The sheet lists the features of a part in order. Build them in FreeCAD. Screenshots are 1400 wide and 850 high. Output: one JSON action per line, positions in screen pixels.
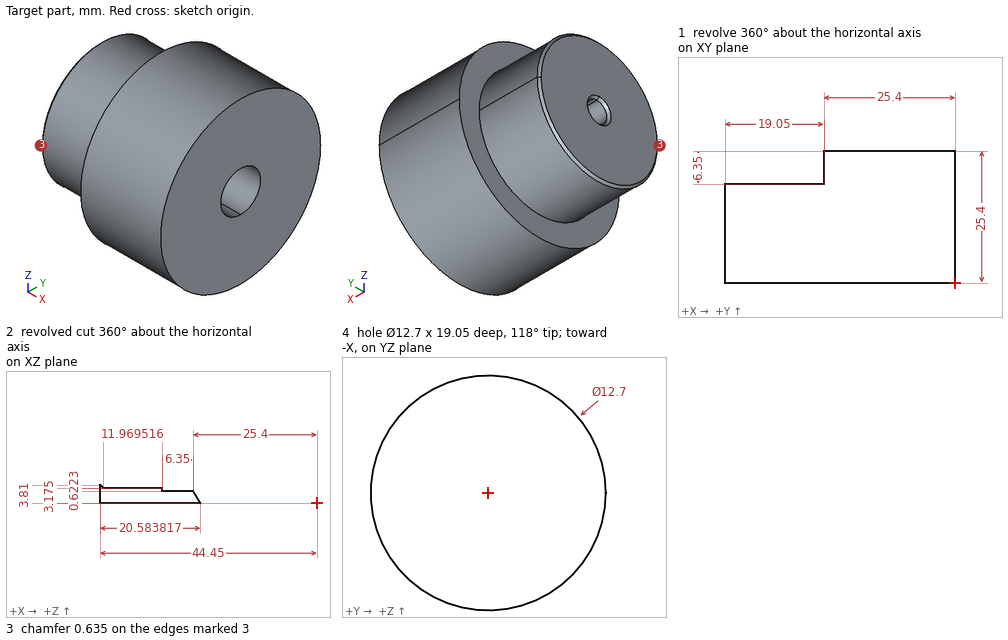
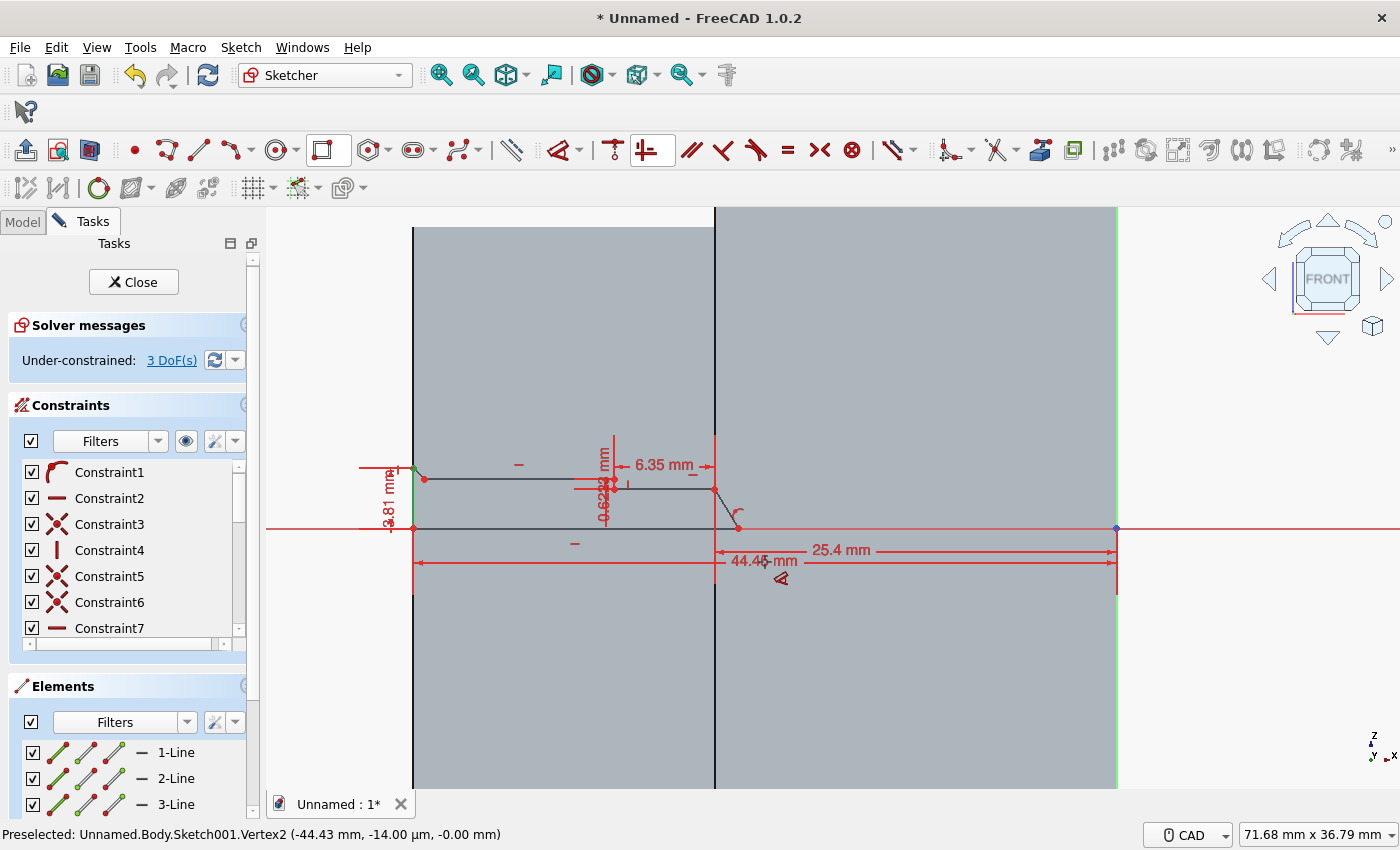
{"action": "left_click", "coordinate": [425, 479]}
{"action": "left_click", "coordinate": [1151, 504]}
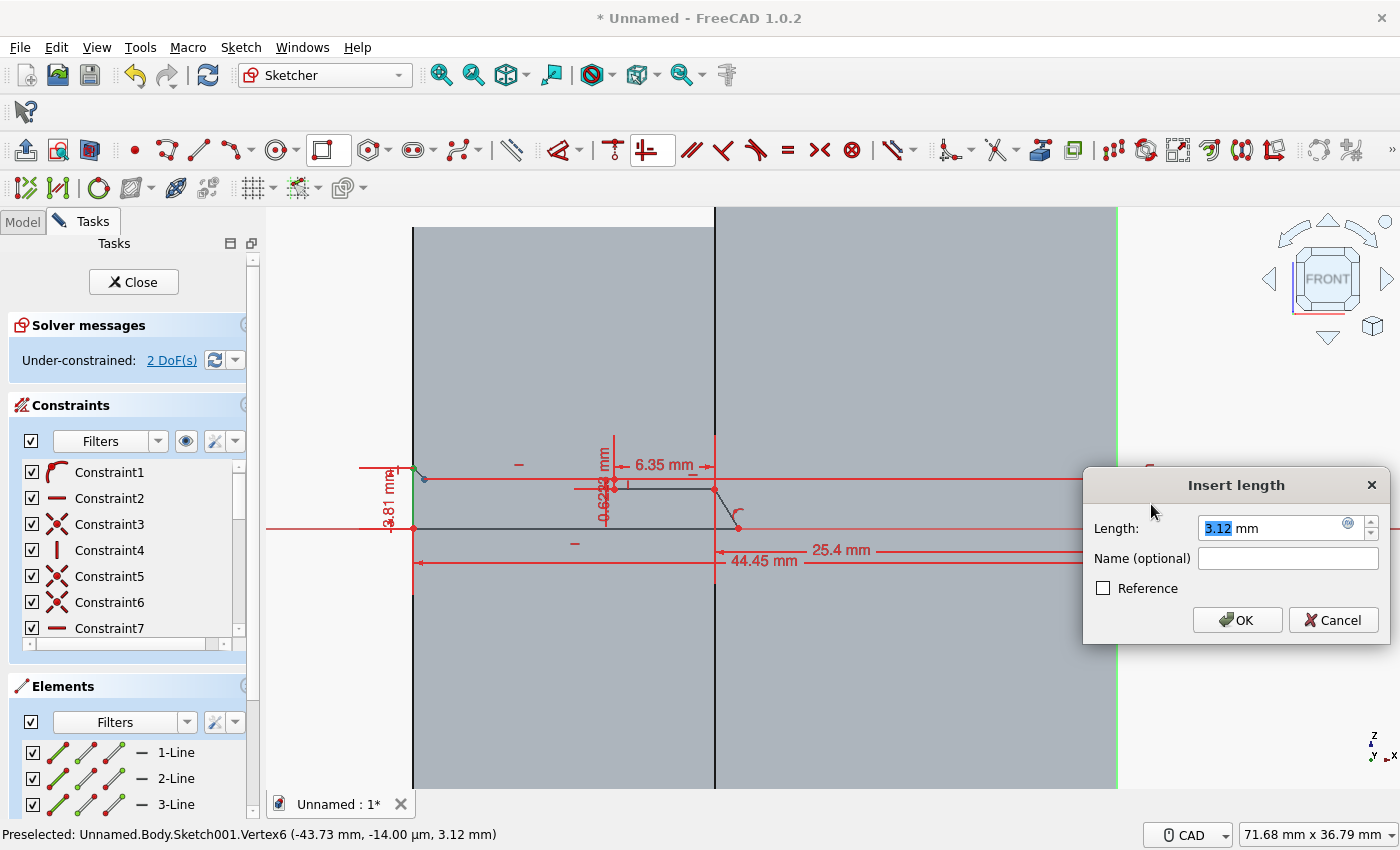
{"action": "type", "text": "3.175"}
{"action": "key", "text": "Return"}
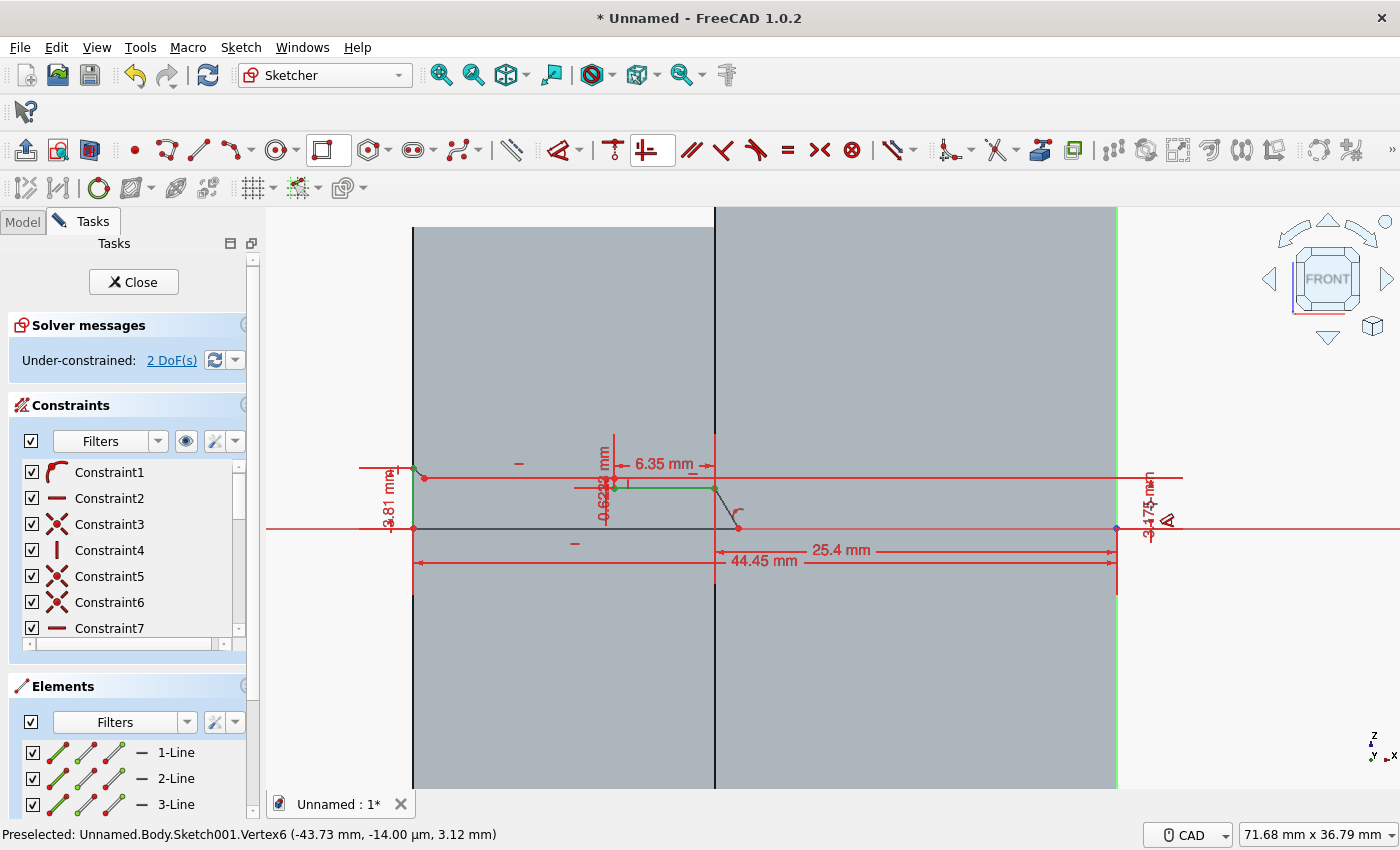
{"action": "left_click", "coordinate": [641, 528]}
{"action": "left_click", "coordinate": [576, 562]}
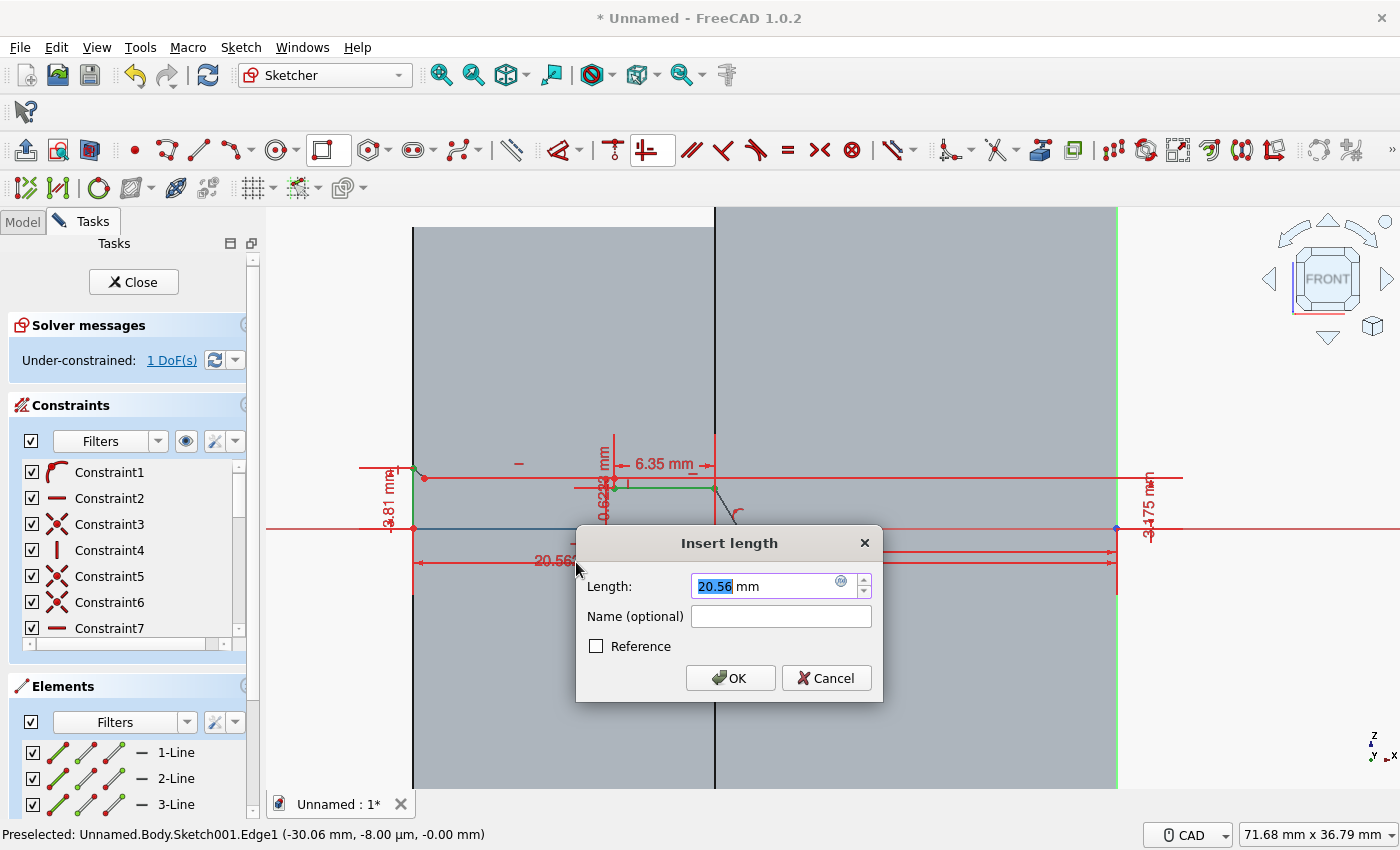
{"action": "type", "text": "20.583817"}
{"action": "key", "text": "Return"}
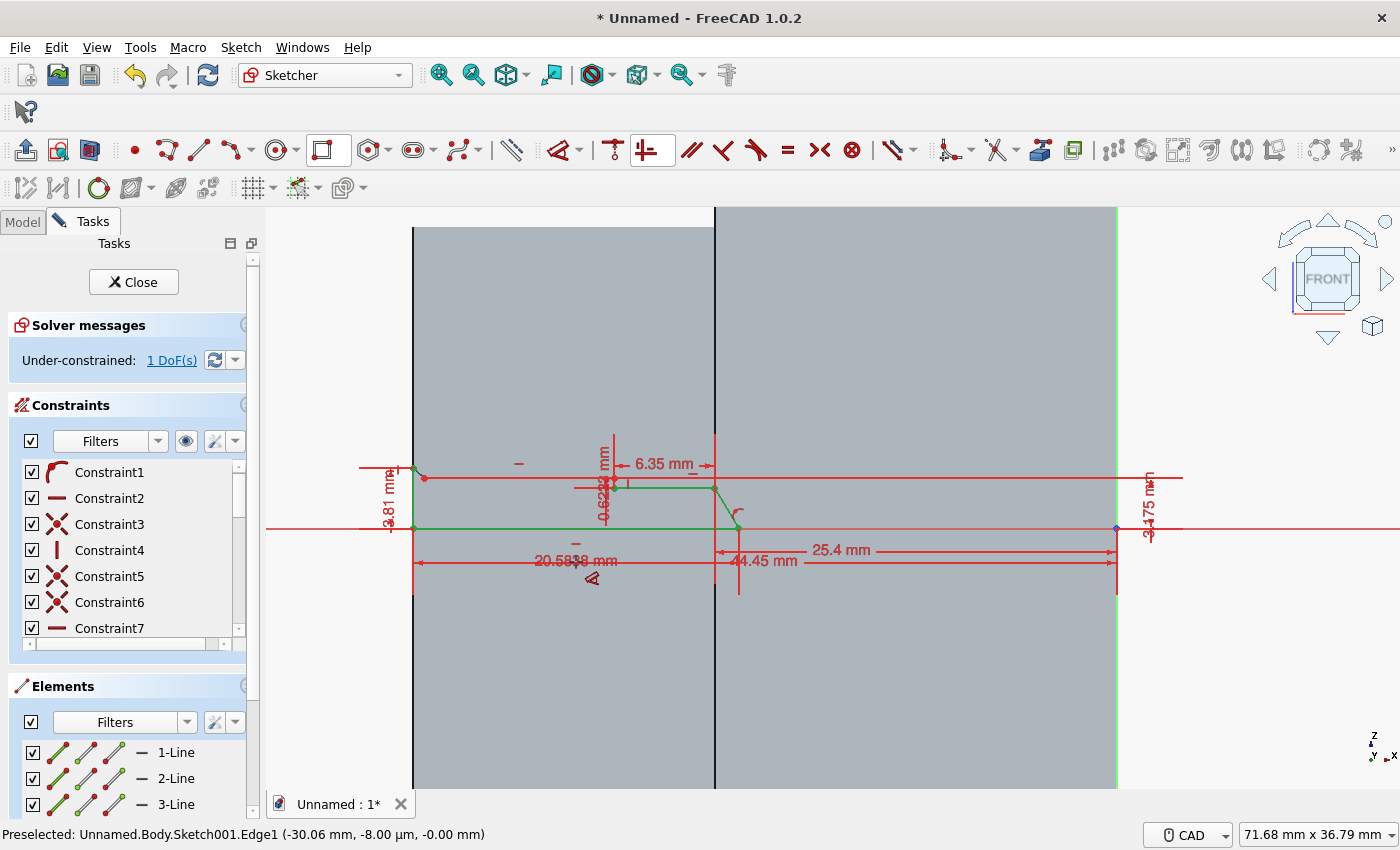
{"action": "left_click", "coordinate": [482, 478]}
{"action": "left_click", "coordinate": [519, 444]}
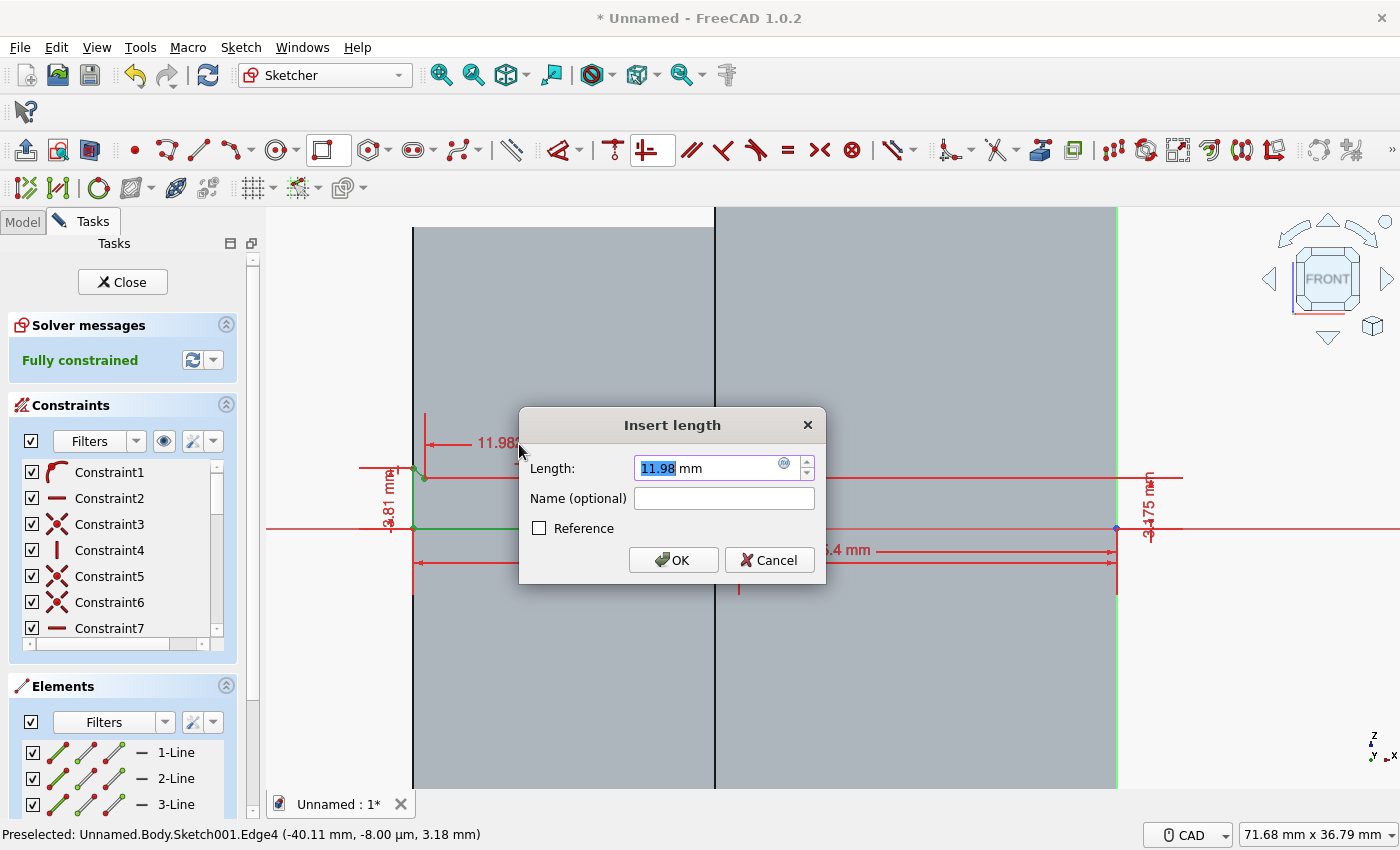
{"action": "type", "text": "11.969516"}
{"action": "key", "text": "Return"}
{"action": "key", "text": "Escape"}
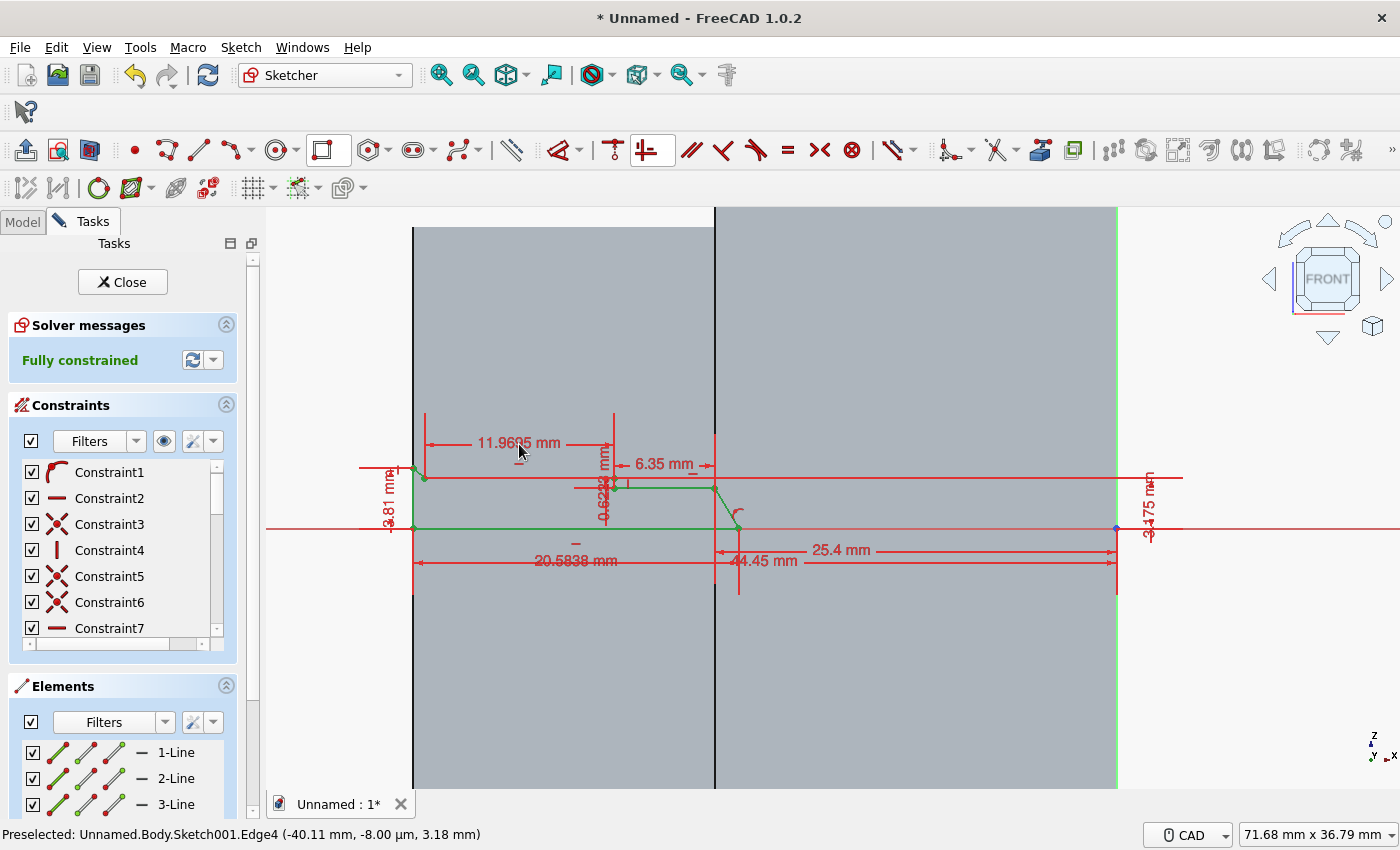
{"action": "left_click", "coordinate": [123, 282]}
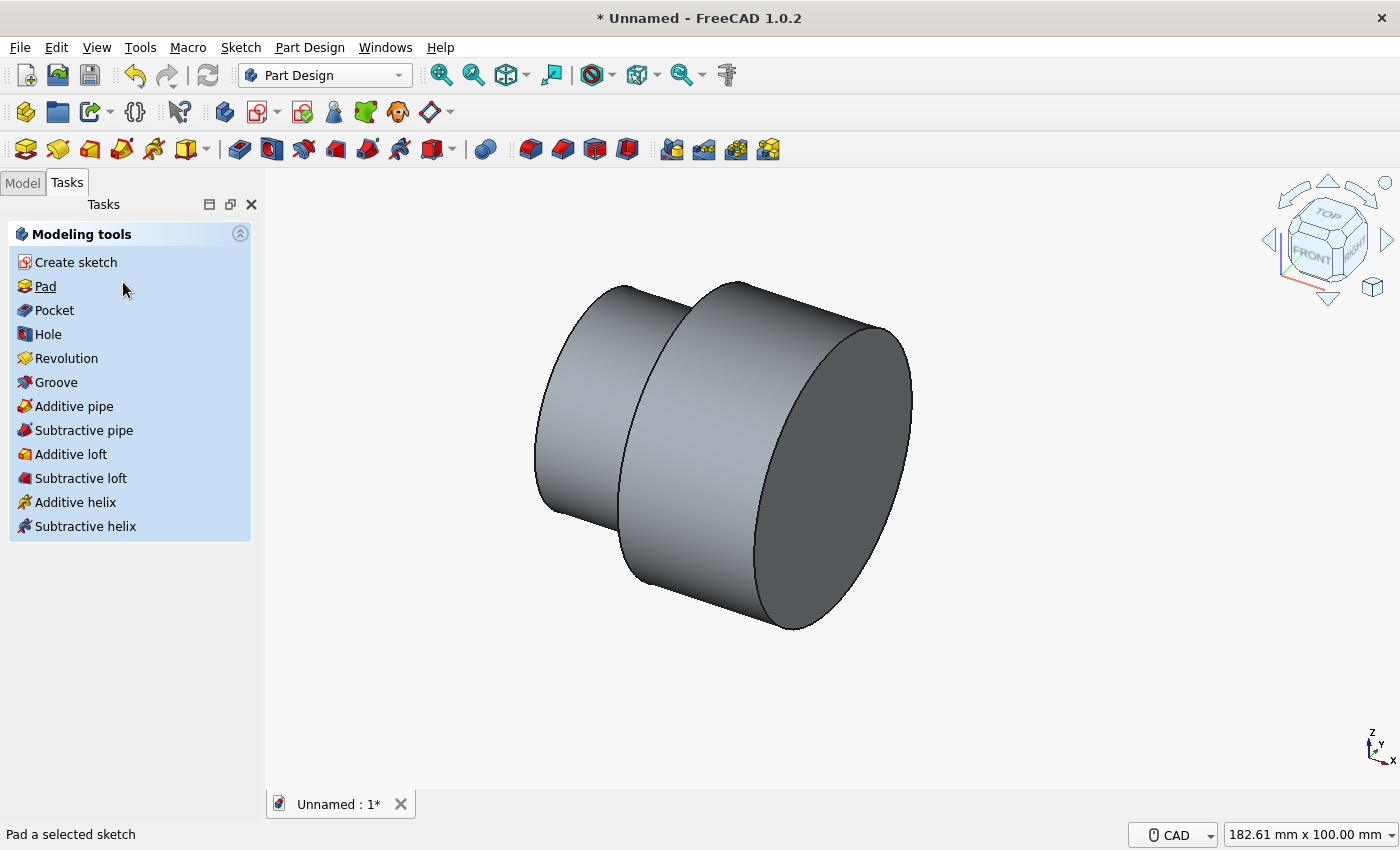
{"action": "left_click", "coordinate": [304, 150]}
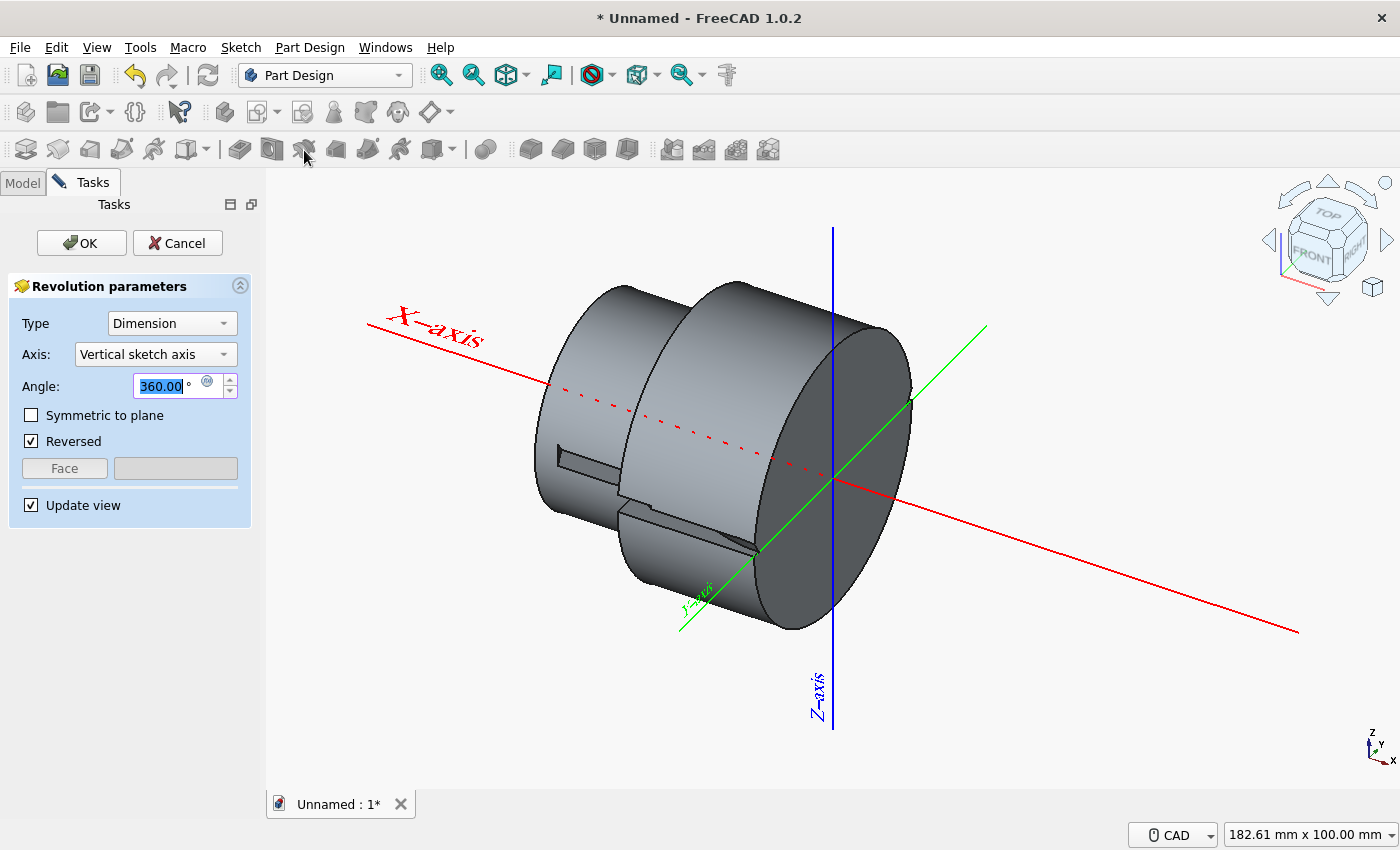
{"action": "left_click", "coordinate": [156, 354]}